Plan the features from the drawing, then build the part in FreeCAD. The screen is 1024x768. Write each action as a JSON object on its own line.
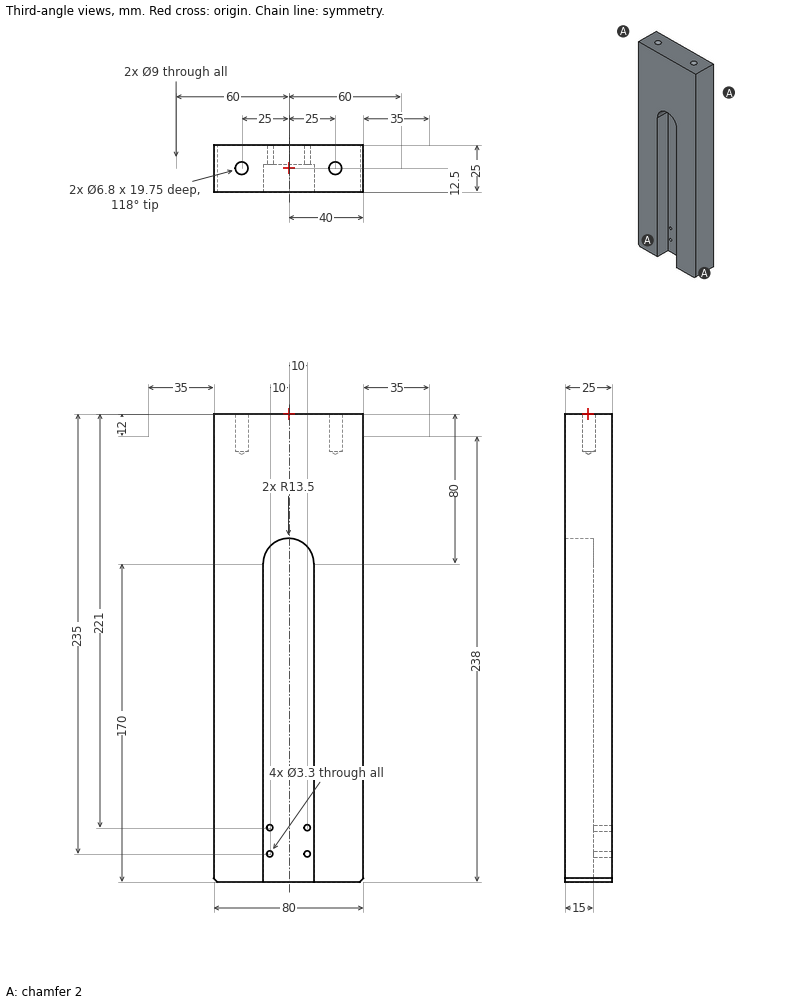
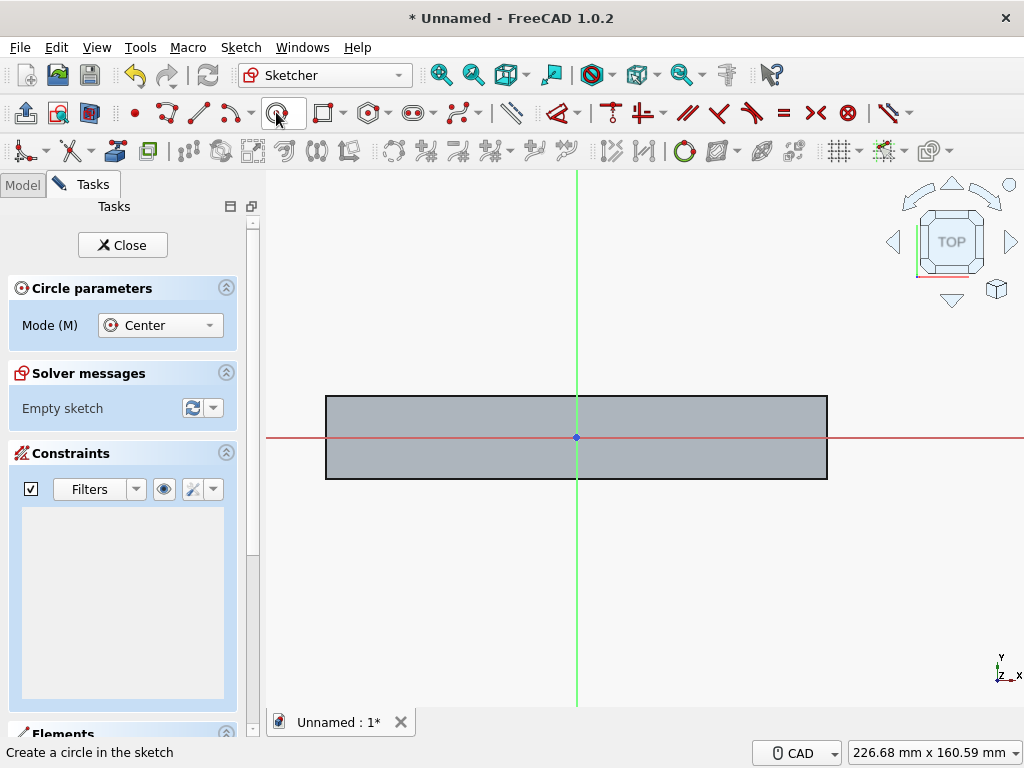
{"action": "scroll", "coordinate": [376, 438], "scroll_direction": "up", "scroll_amount": 3}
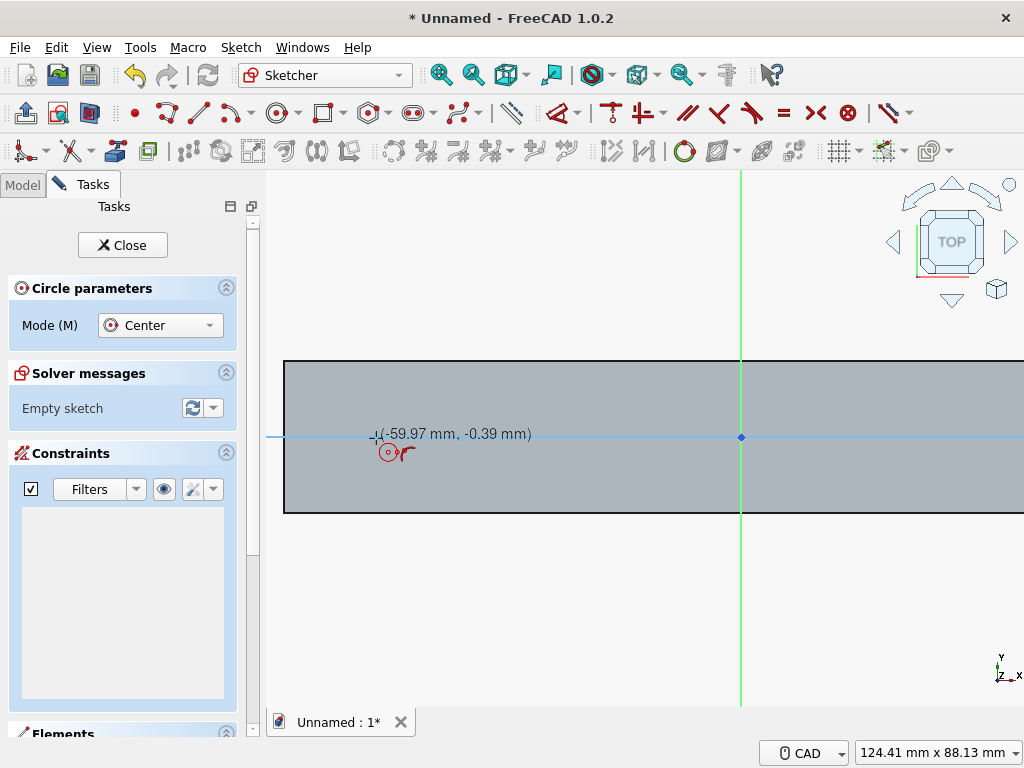
{"action": "left_click", "coordinate": [376, 437]}
{"action": "left_click", "coordinate": [395, 418]}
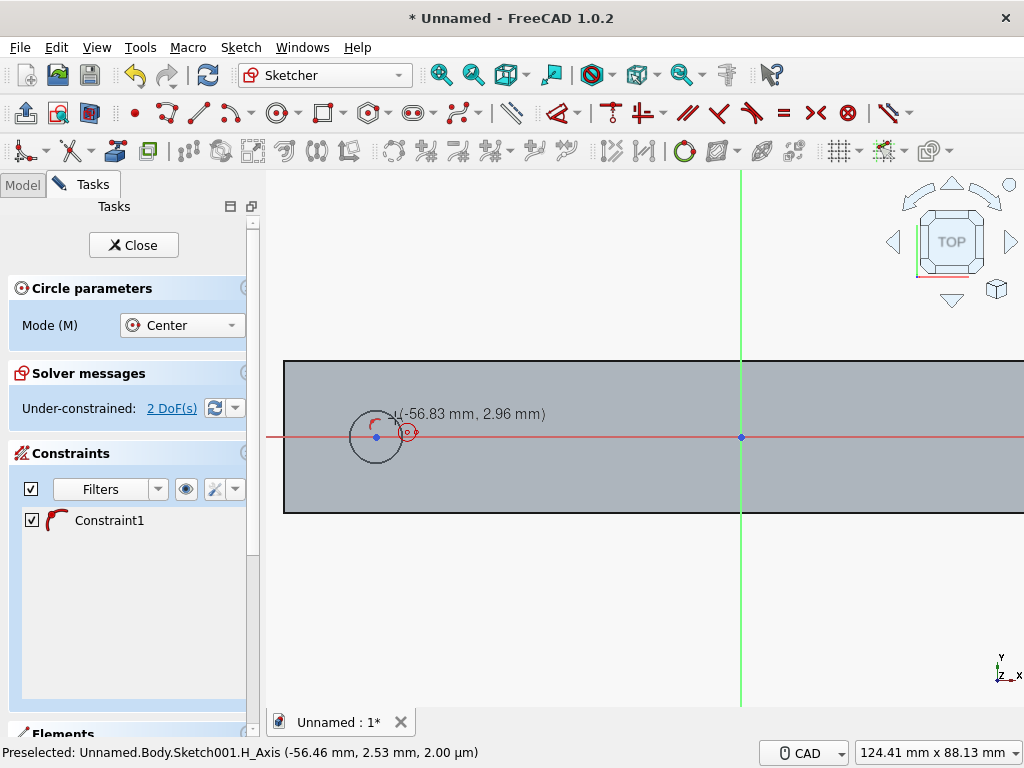
{"action": "scroll", "coordinate": [376, 440], "scroll_direction": "down", "scroll_amount": 3}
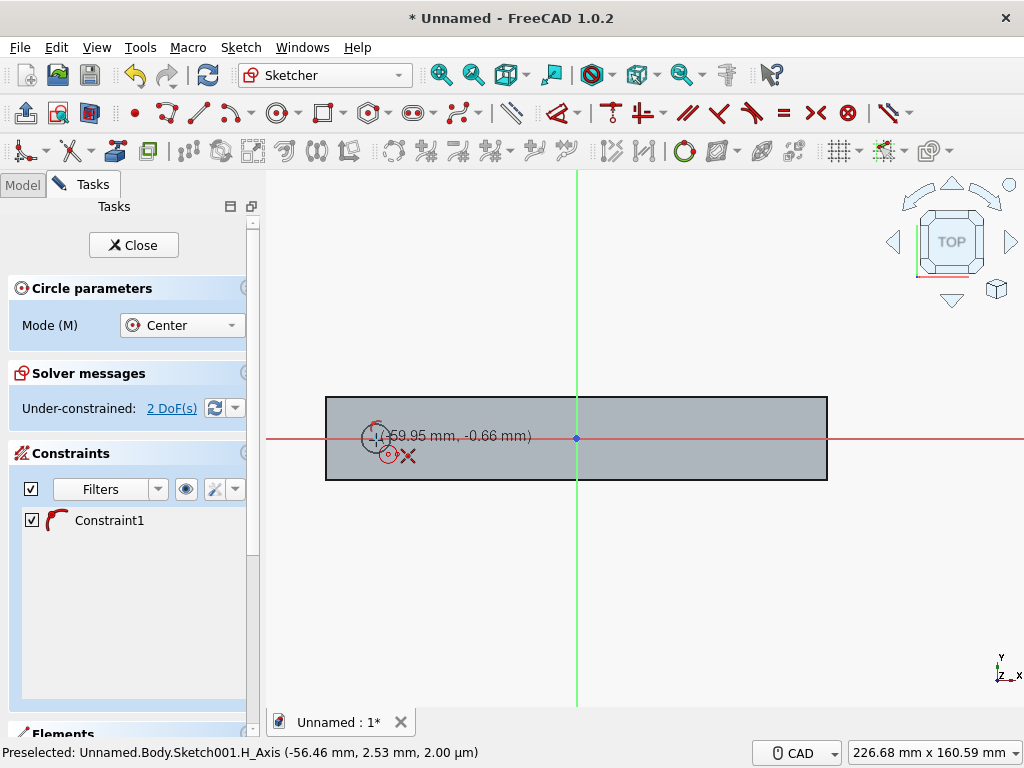
{"action": "scroll", "coordinate": [777, 439], "scroll_direction": "up", "scroll_amount": 3}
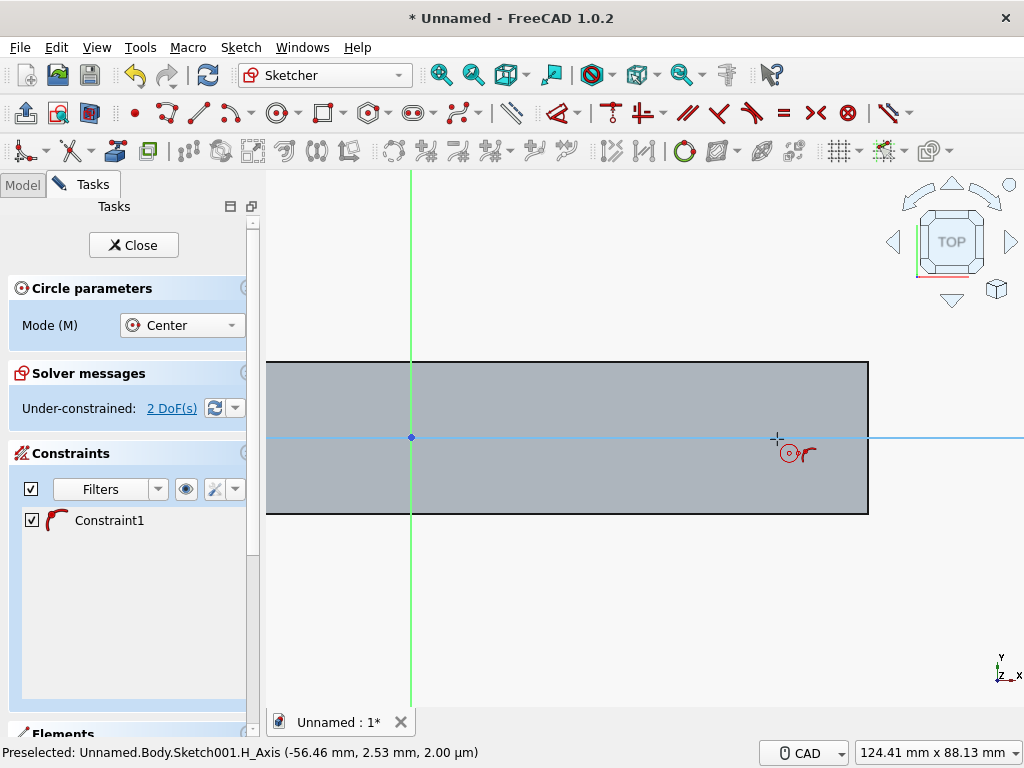
{"action": "left_click", "coordinate": [777, 438]}
{"action": "left_click", "coordinate": [796, 418]}
{"action": "key", "text": "Escape"}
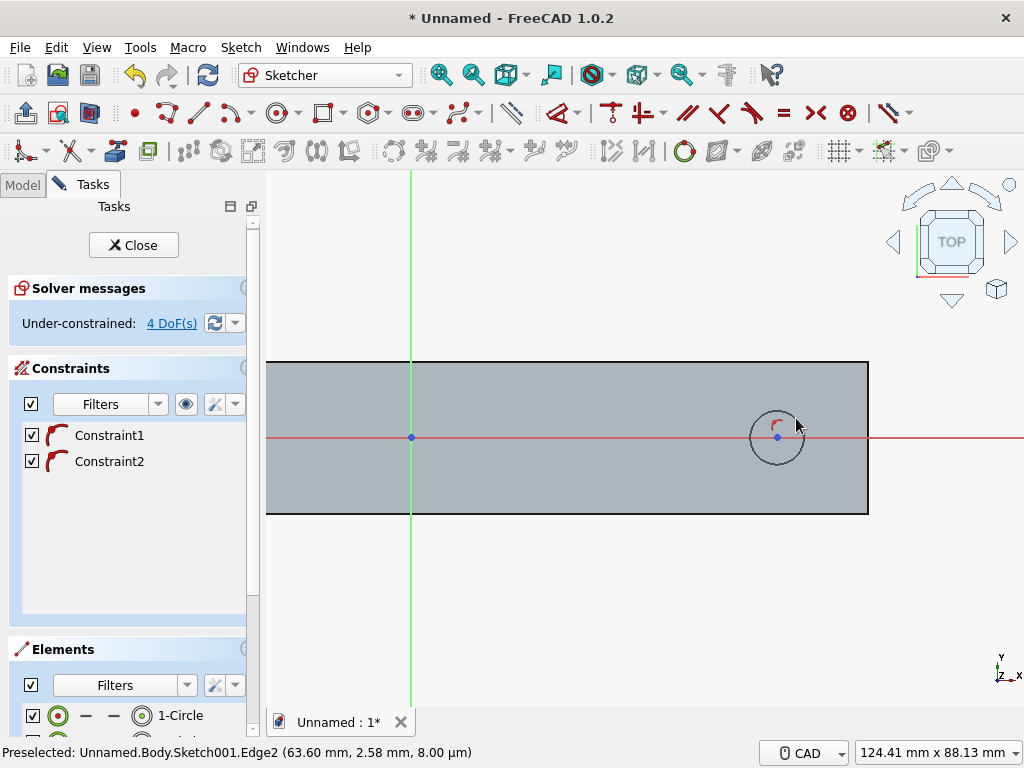
{"action": "scroll", "coordinate": [778, 439], "scroll_direction": "down", "scroll_amount": 3}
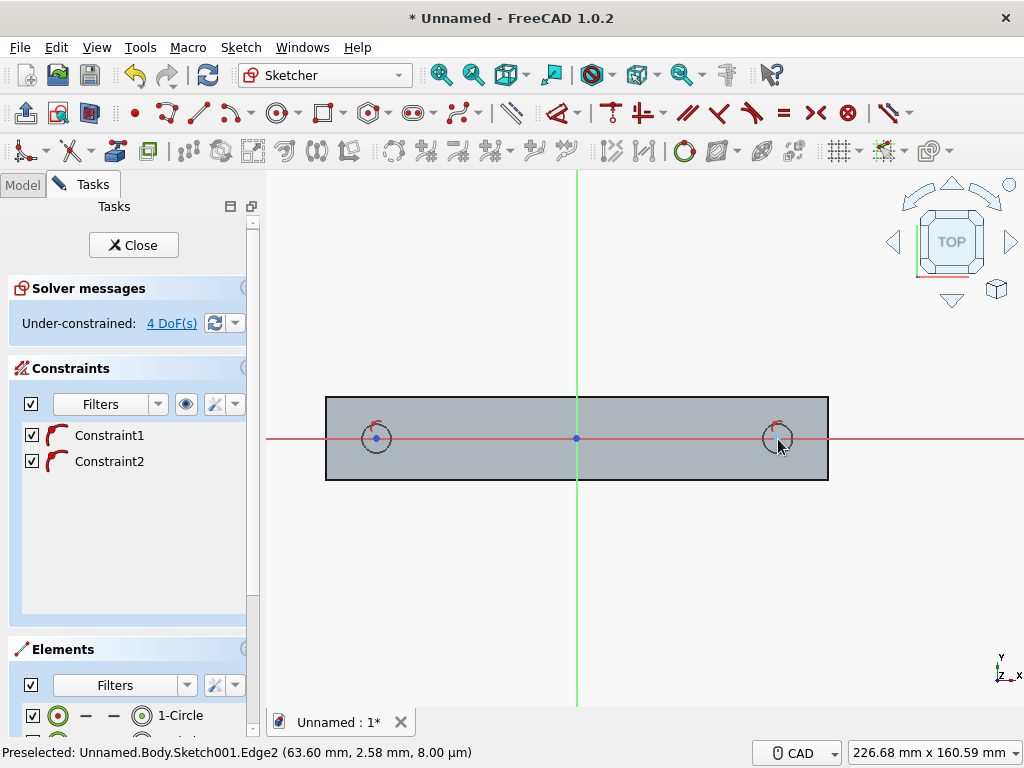
{"action": "scroll", "coordinate": [387, 428], "scroll_direction": "up", "scroll_amount": 2}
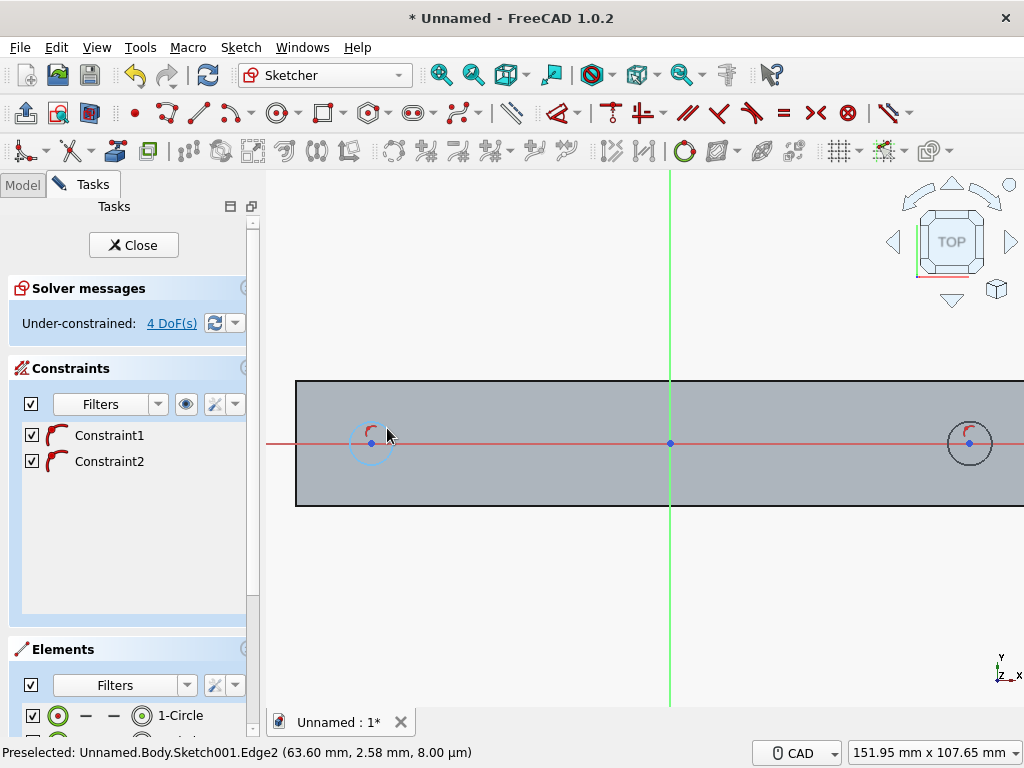
{"action": "left_click", "coordinate": [386, 428]}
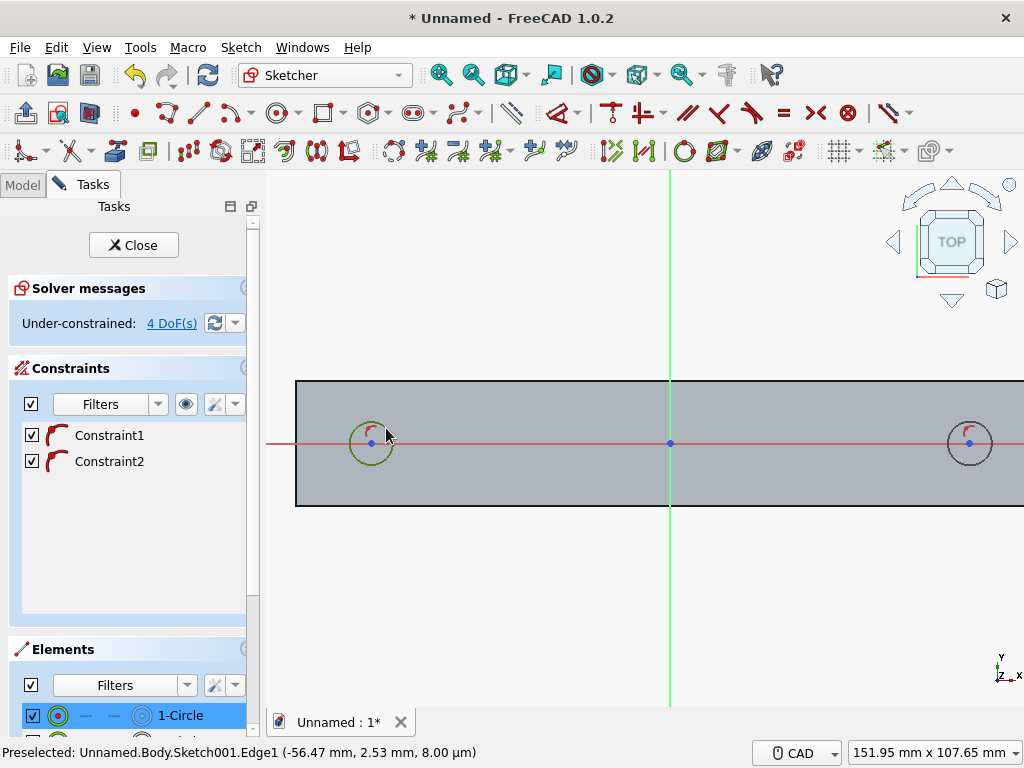
{"action": "scroll", "coordinate": [386, 428], "scroll_direction": "down", "scroll_amount": 2}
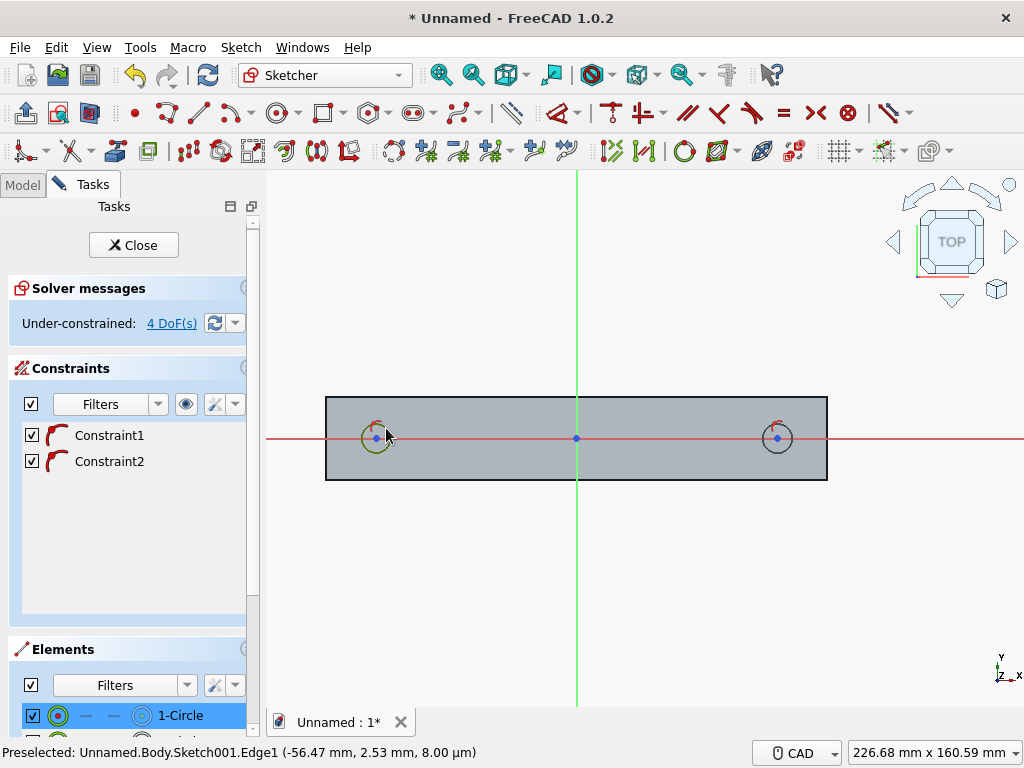
{"action": "scroll", "coordinate": [788, 428], "scroll_direction": "up", "scroll_amount": 2}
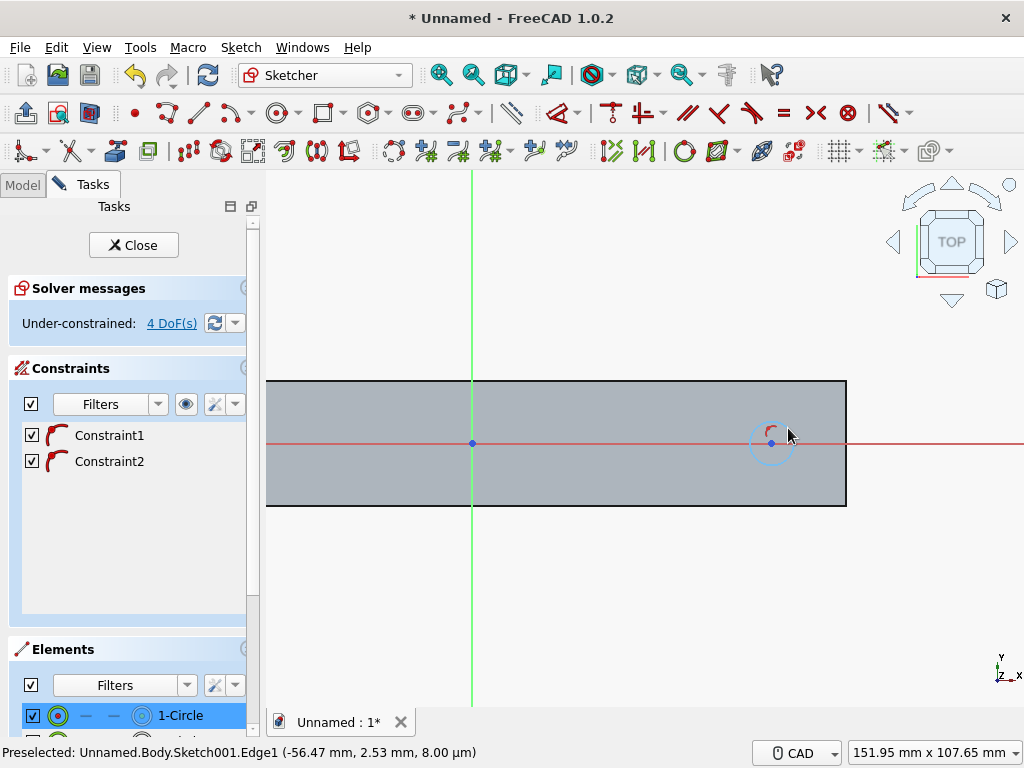
{"action": "left_click", "coordinate": [787, 428]}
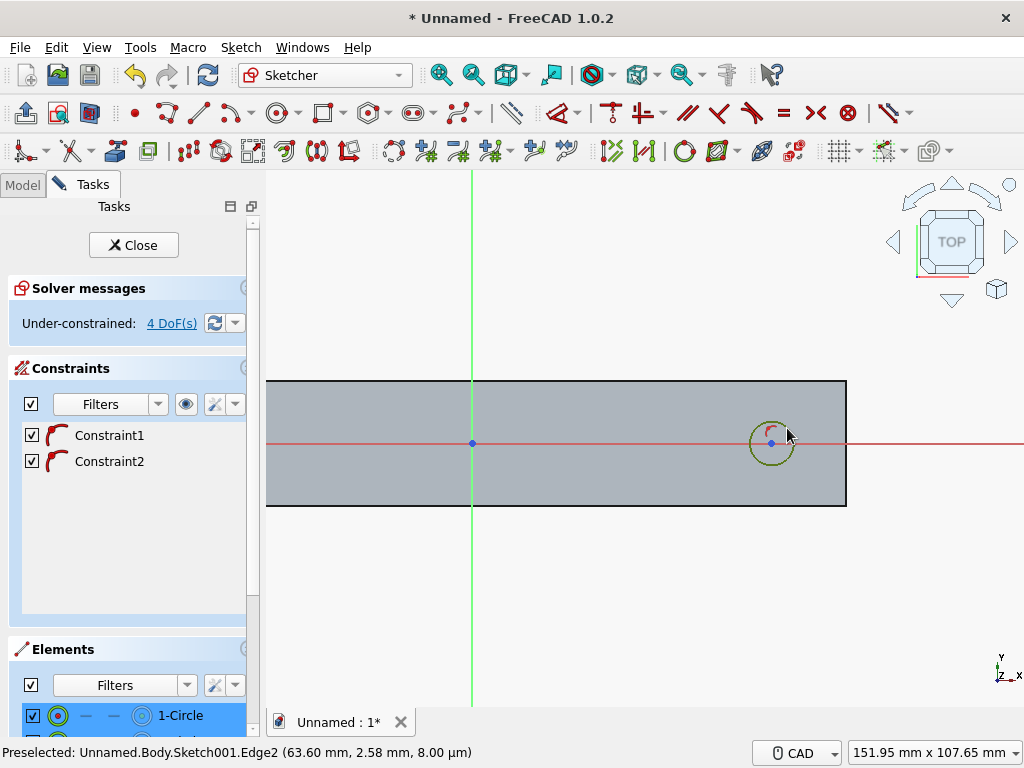
{"action": "left_click", "coordinate": [784, 114]}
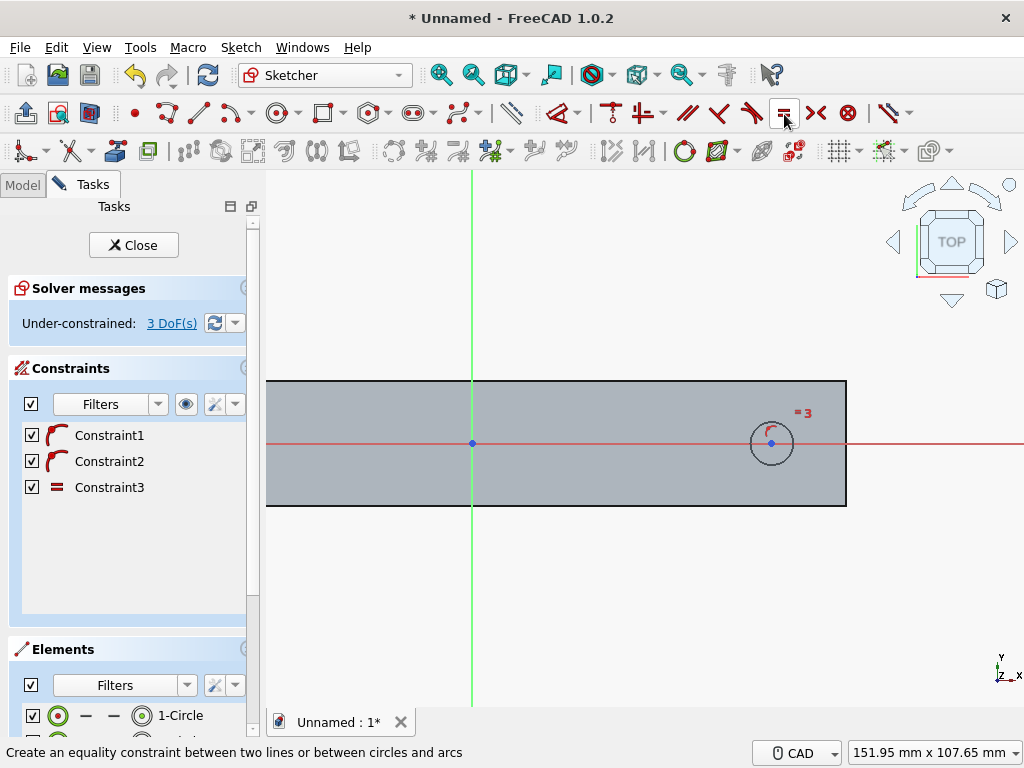
{"action": "left_click", "coordinate": [558, 114]}